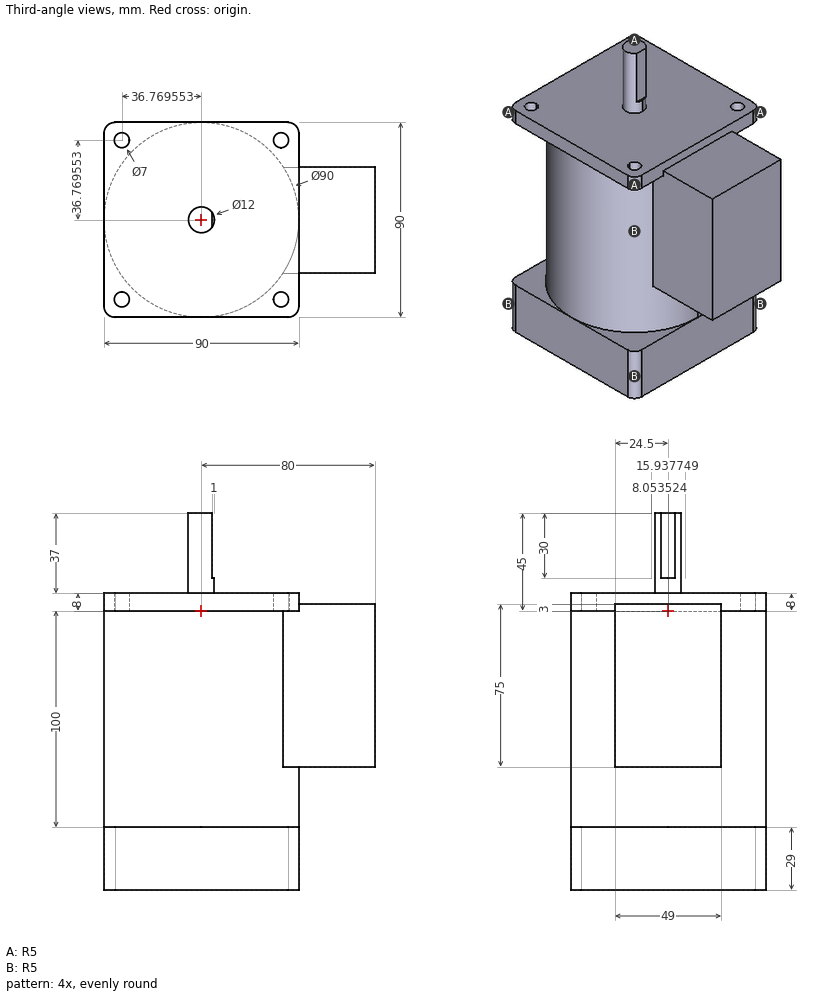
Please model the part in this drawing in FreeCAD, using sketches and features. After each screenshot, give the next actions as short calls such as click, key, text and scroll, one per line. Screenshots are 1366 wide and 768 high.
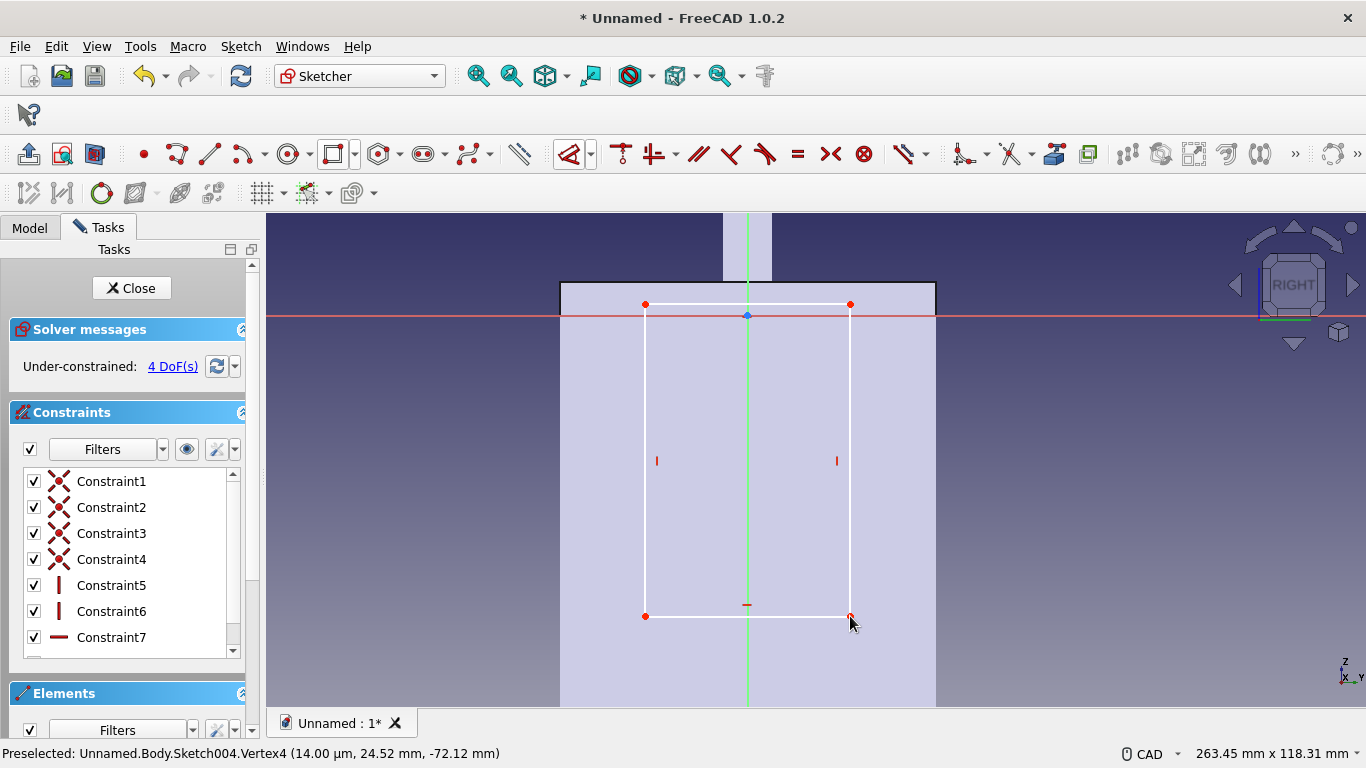
click(645, 398)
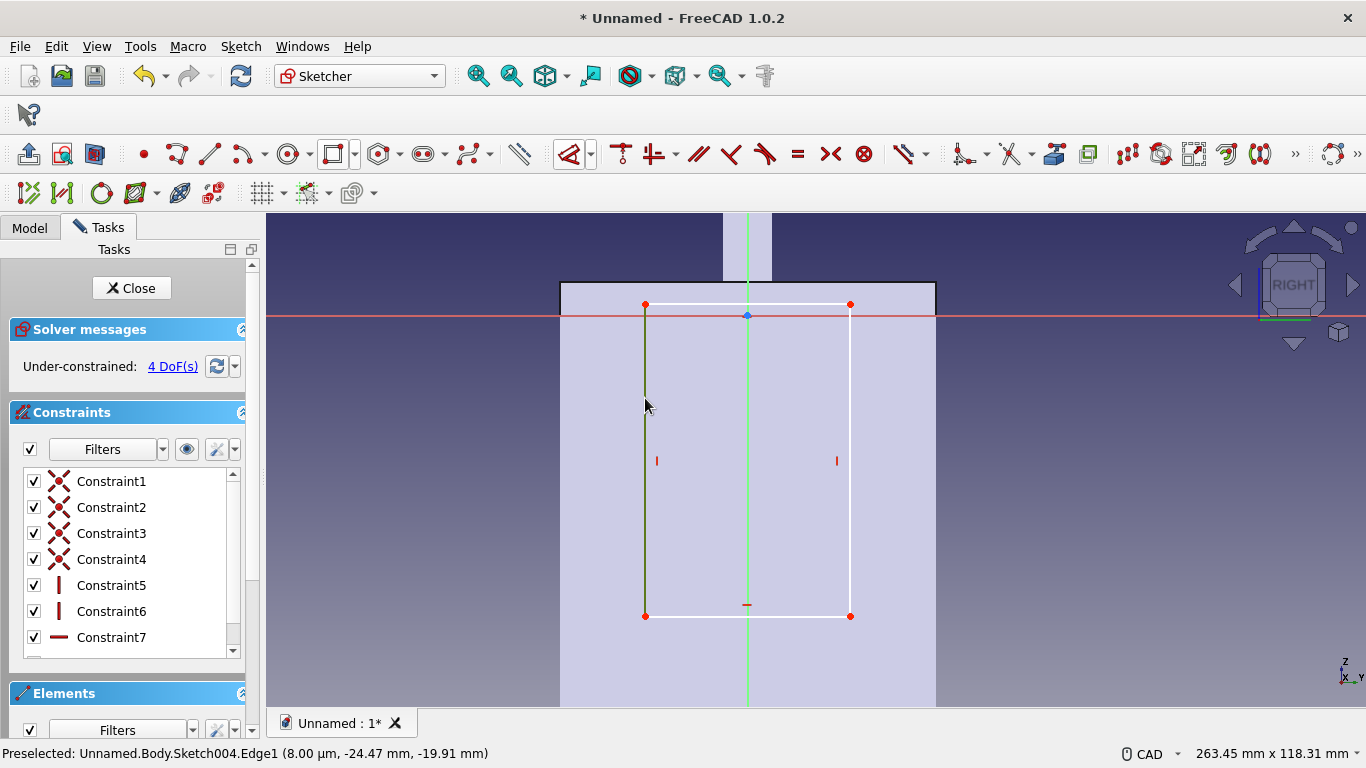
click(590, 154)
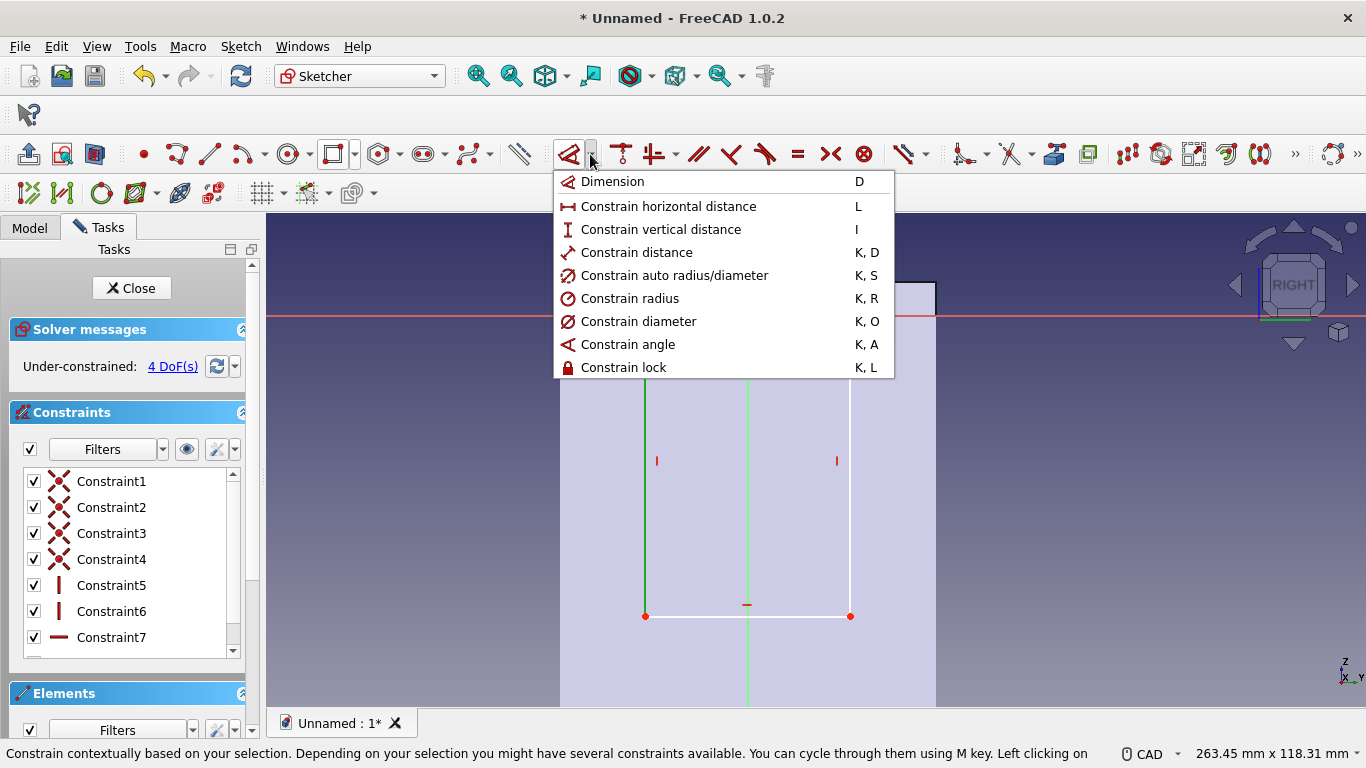
click(724, 230)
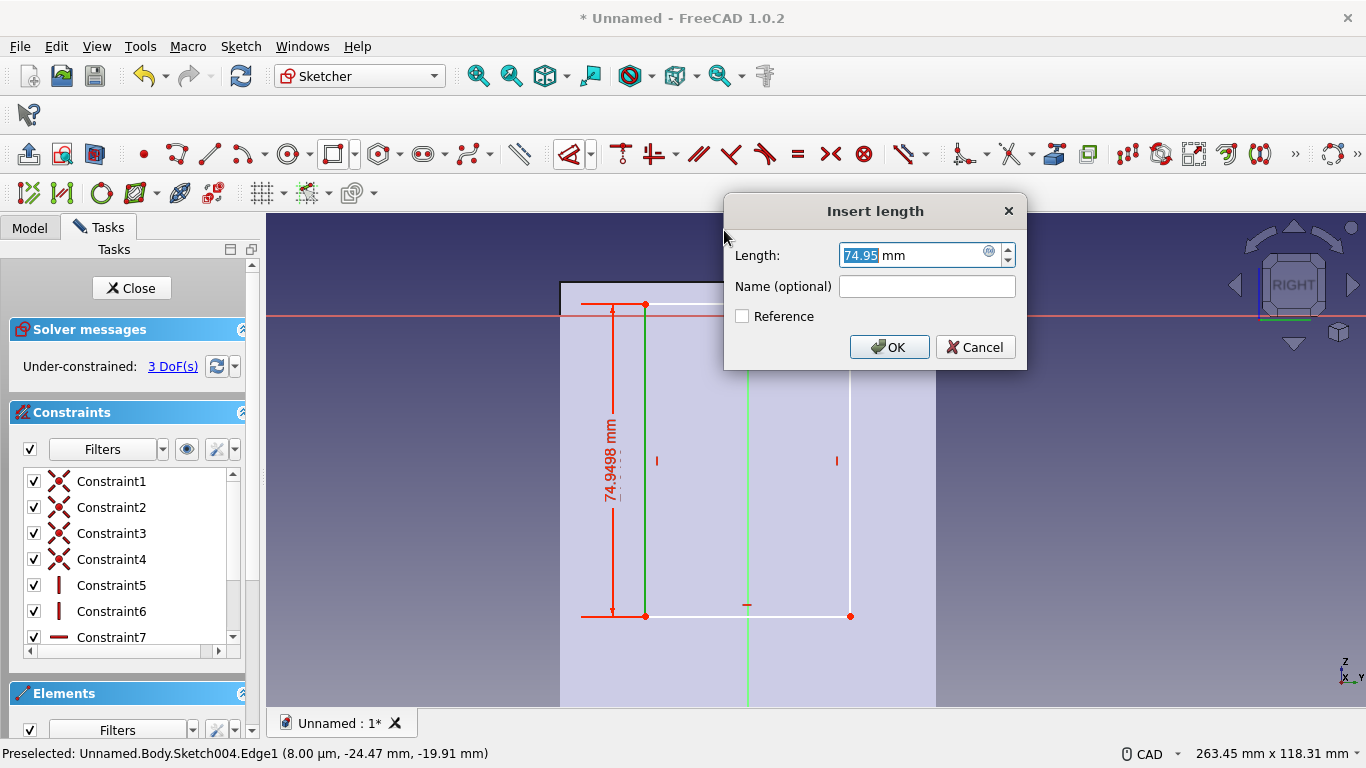
text(75)
key(Return)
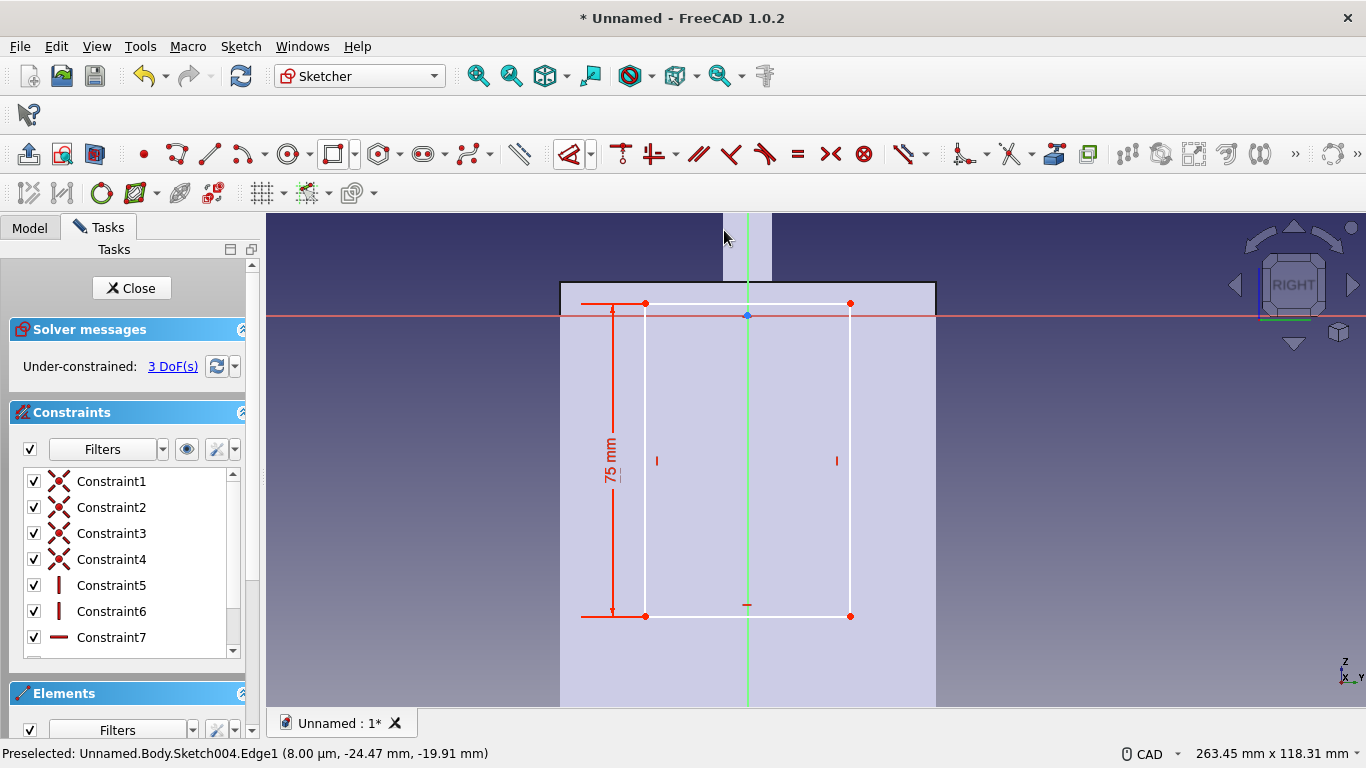
click(707, 617)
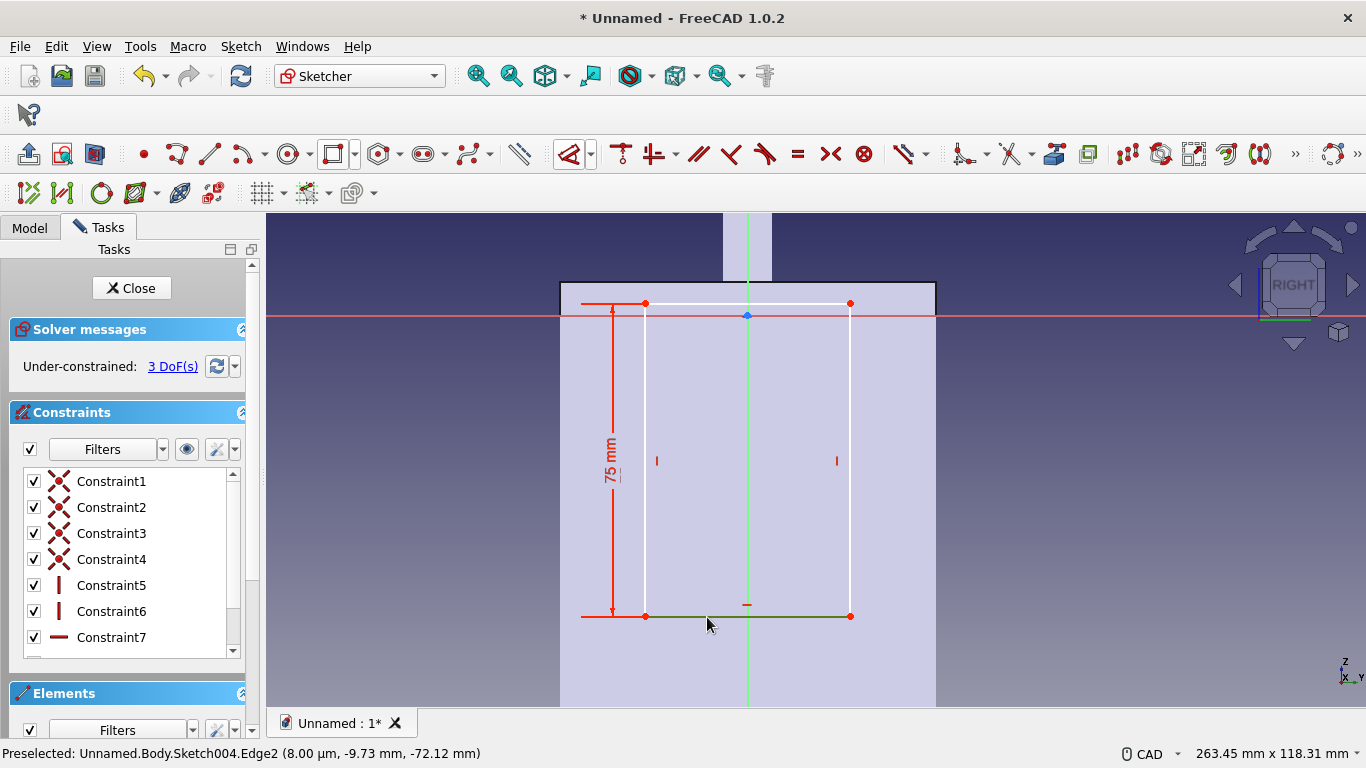
click(590, 154)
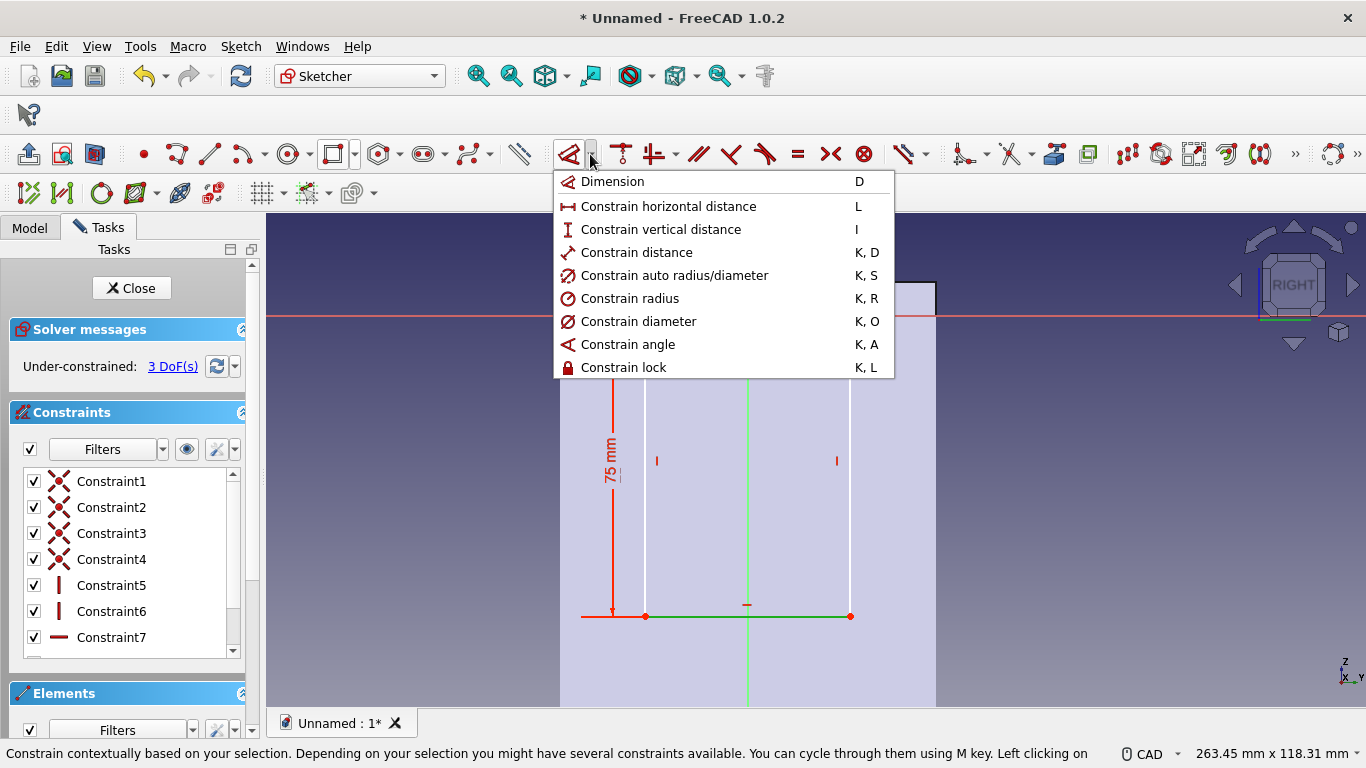
click(724, 206)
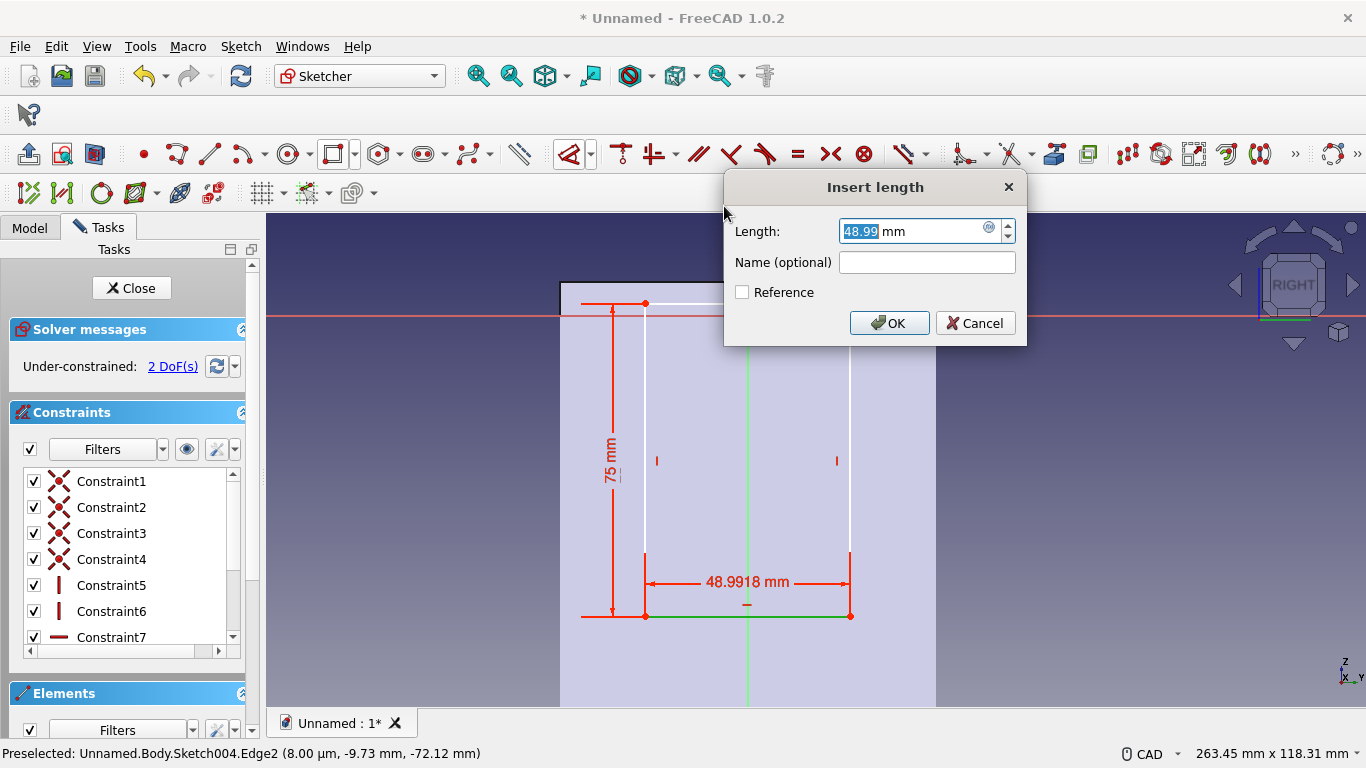
text(49)
key(Return)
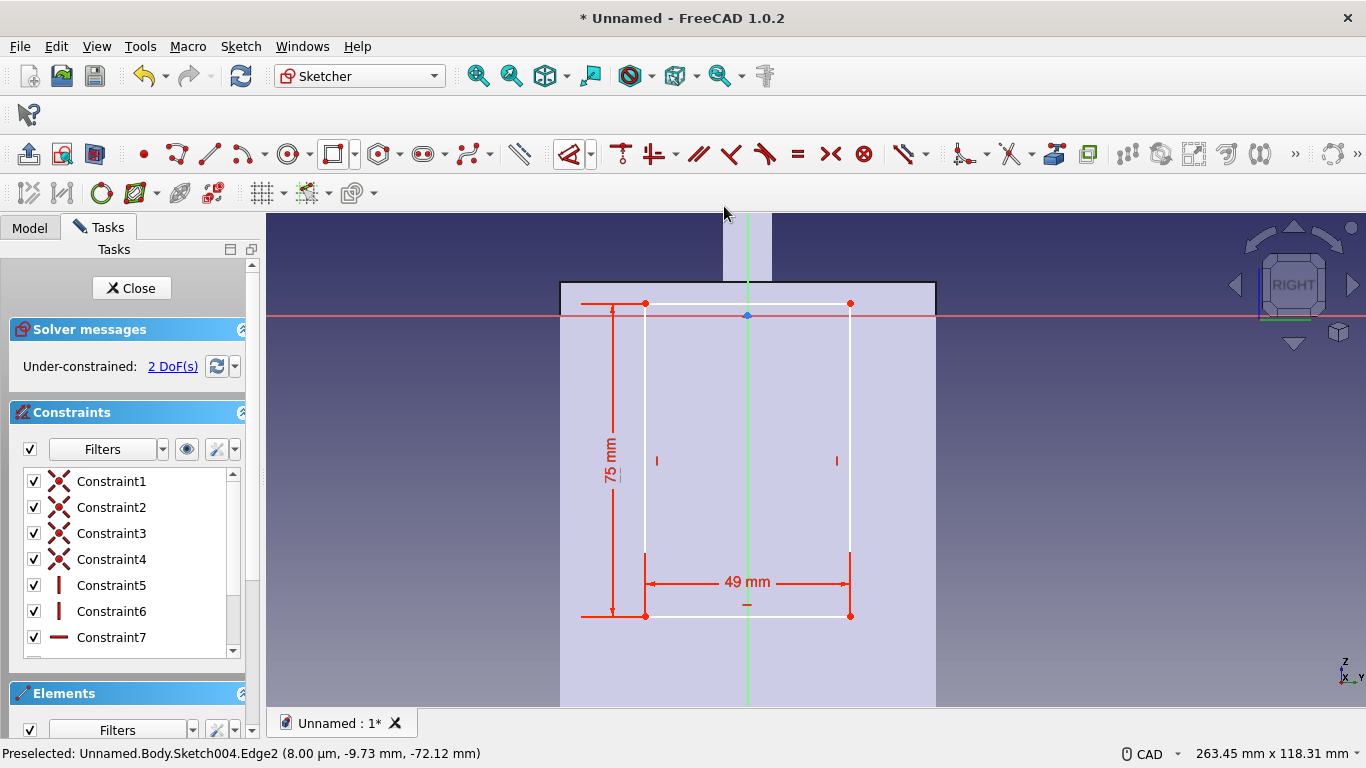
scroll(645, 304, up, 6)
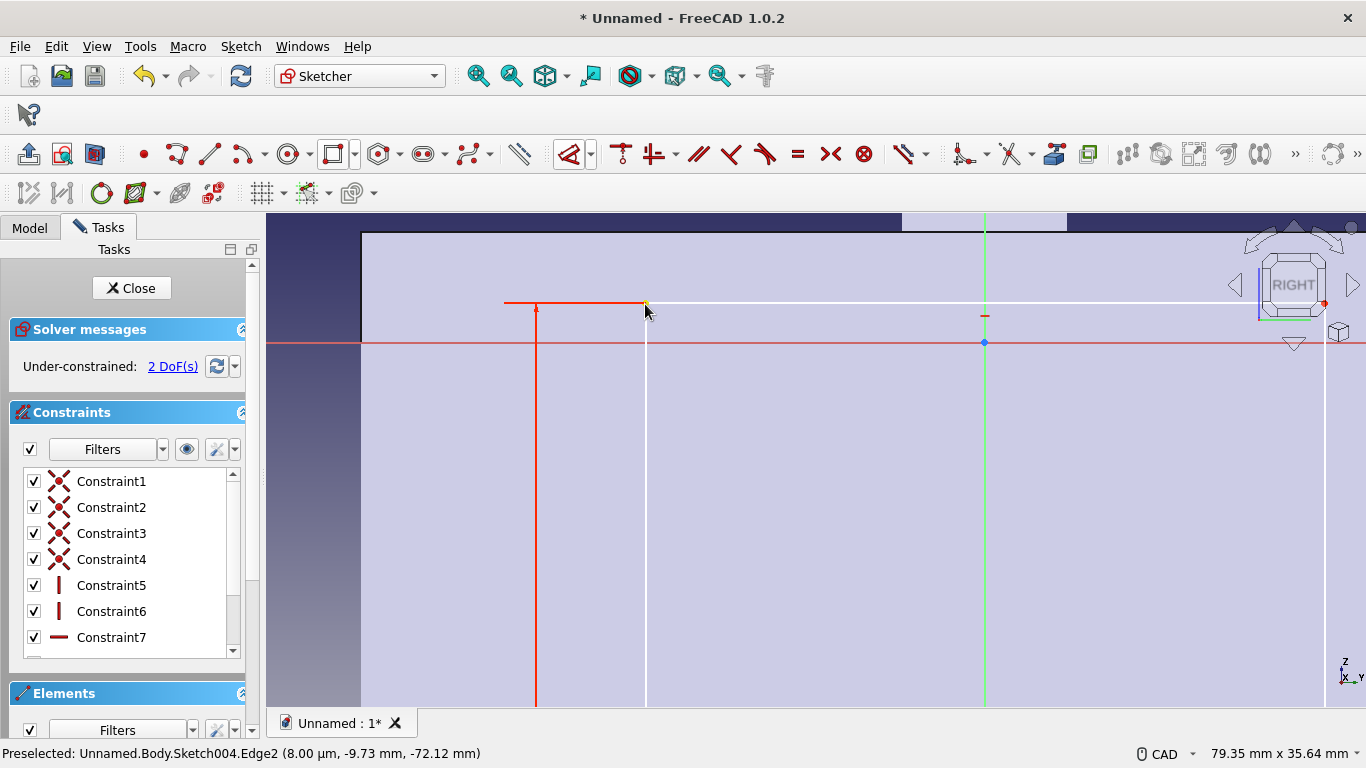
click(646, 303)